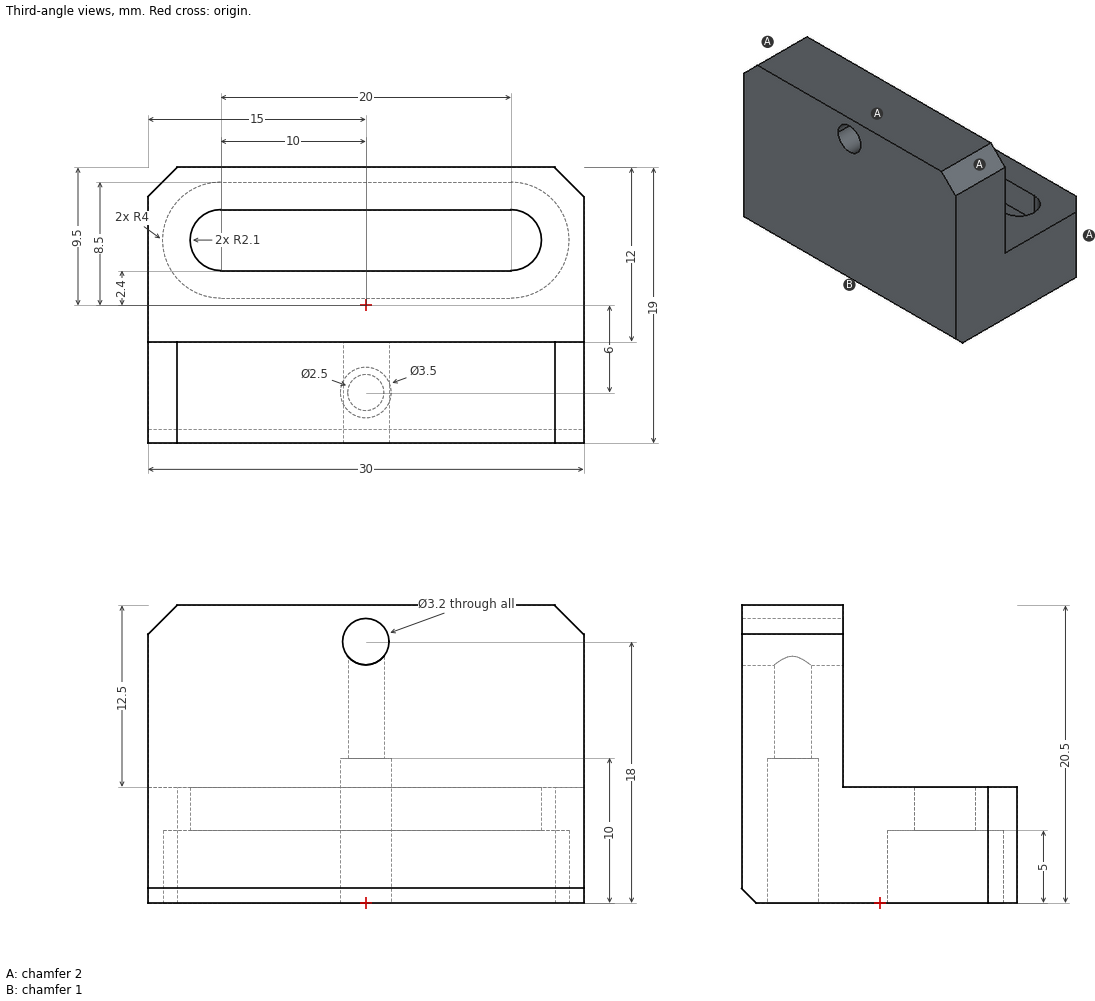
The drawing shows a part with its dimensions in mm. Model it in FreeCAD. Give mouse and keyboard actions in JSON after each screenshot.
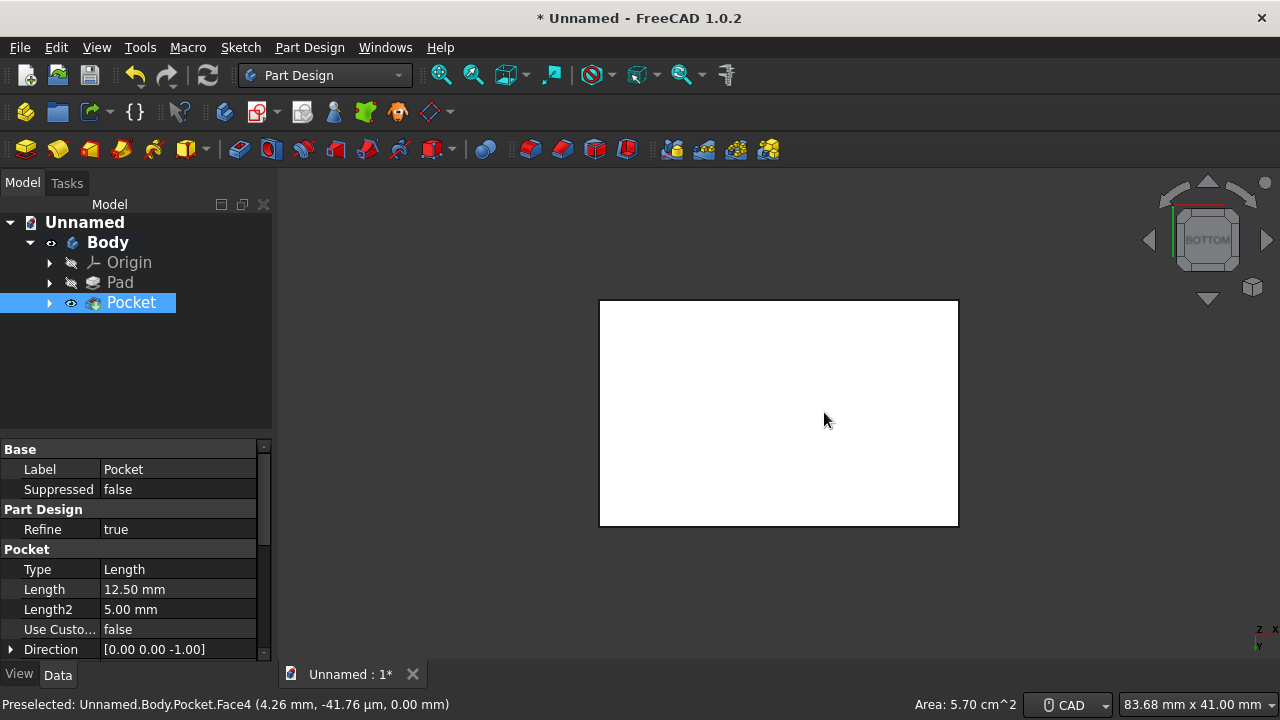
{"action": "left_click", "coordinate": [258, 112]}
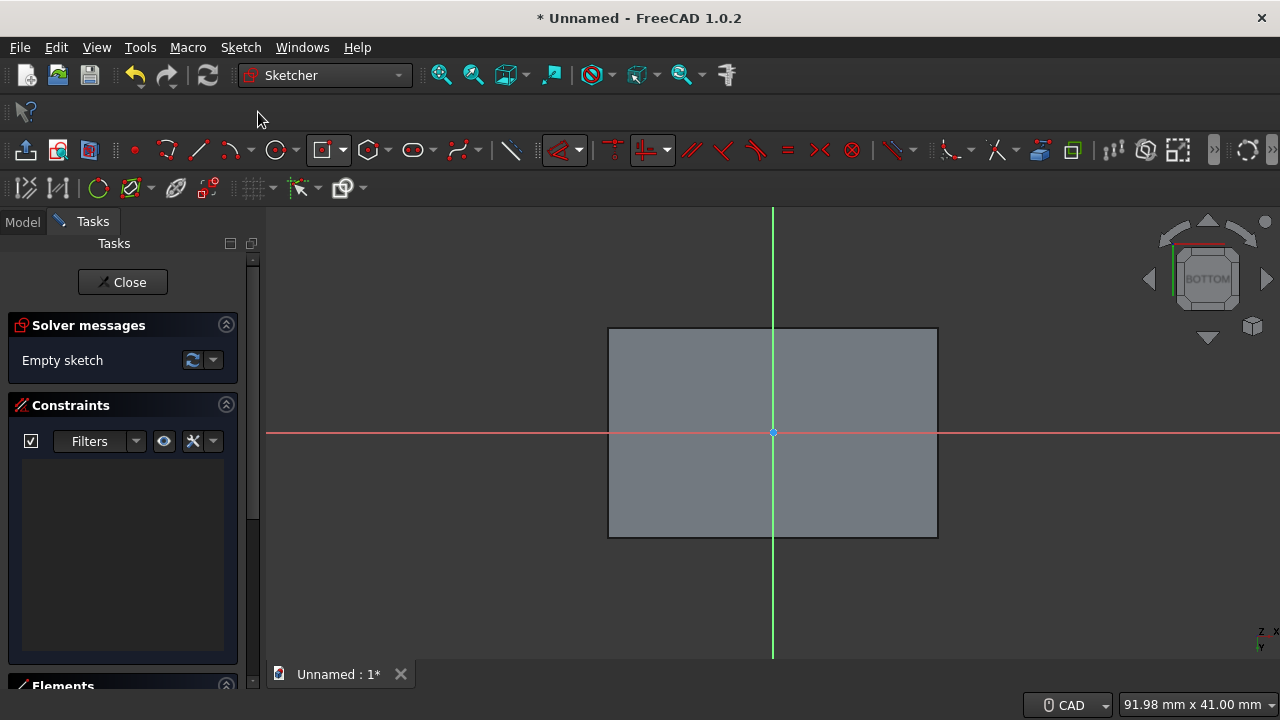
{"action": "scroll", "coordinate": [829, 499], "scroll_direction": "up", "scroll_amount": 4}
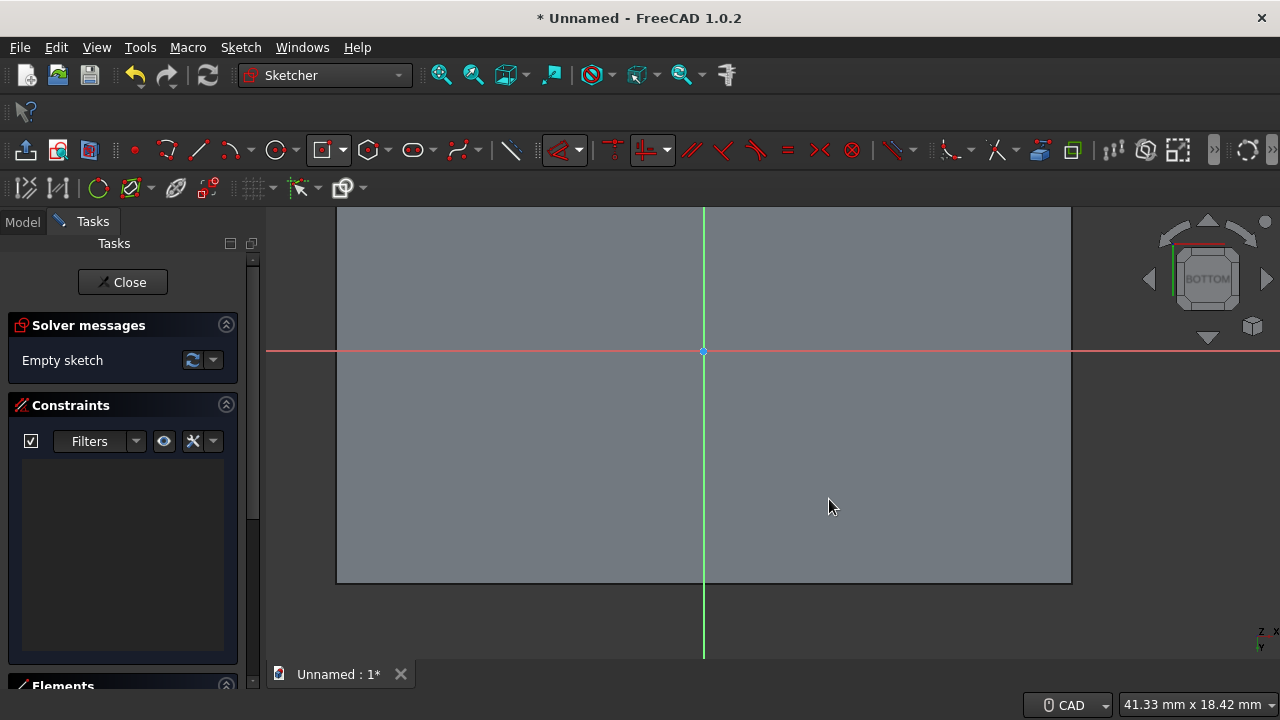
{"action": "left_click", "coordinate": [414, 150]}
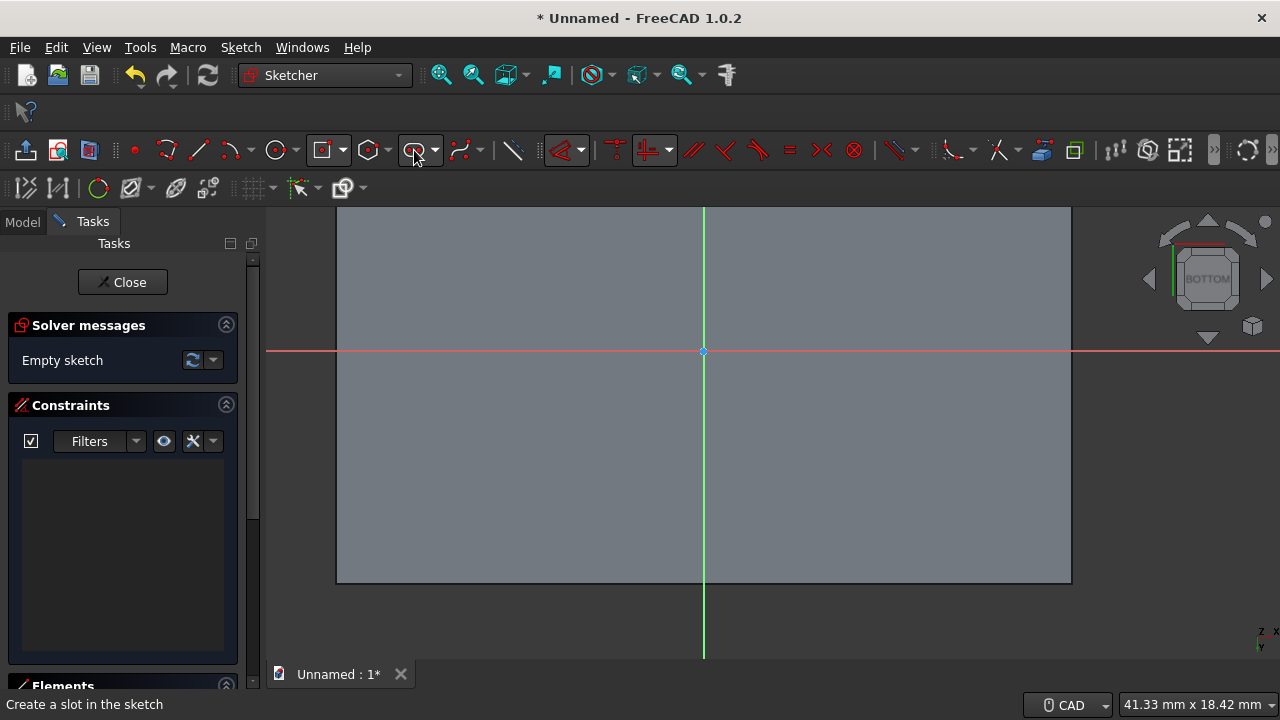
{"action": "left_click", "coordinate": [458, 462]}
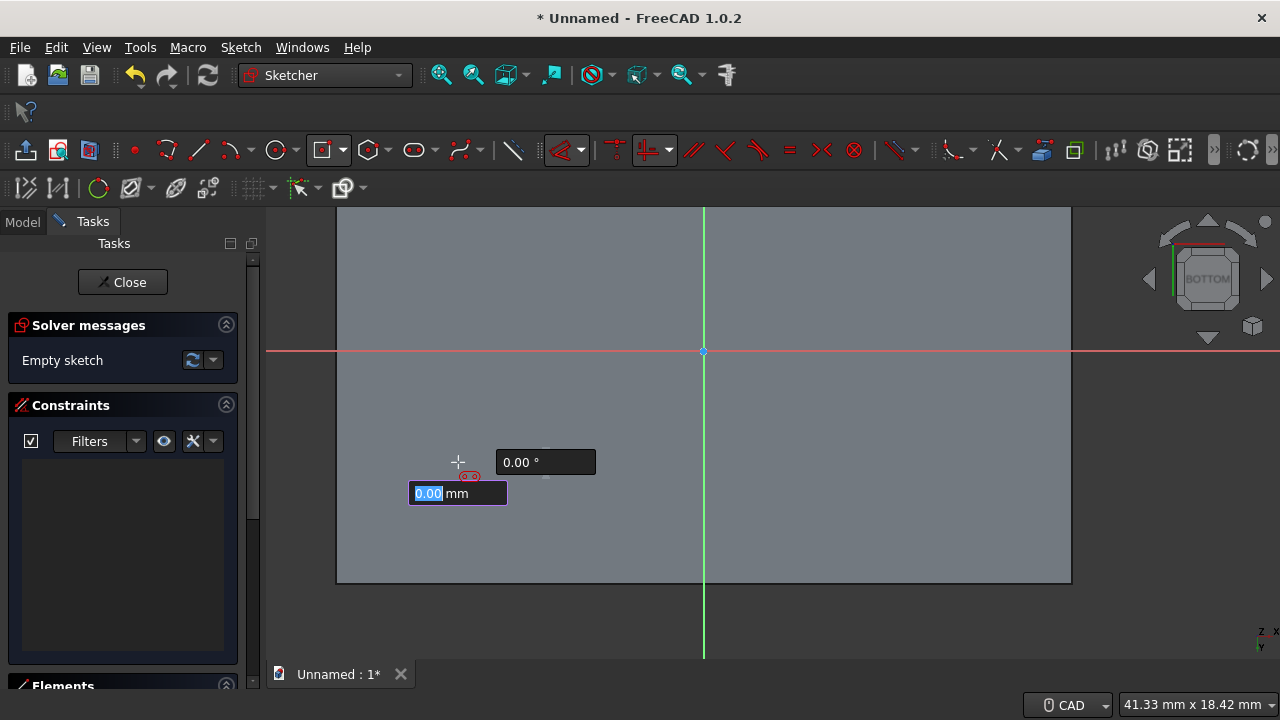
{"action": "left_click", "coordinate": [949, 462]}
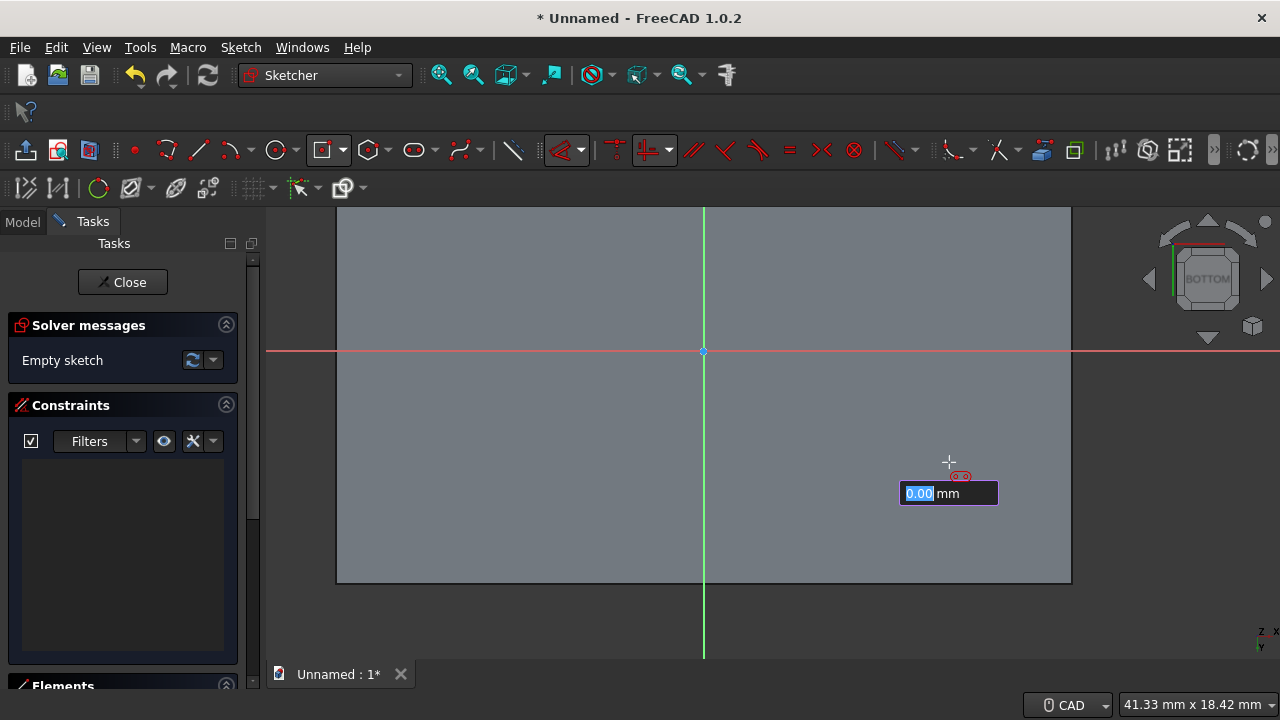
{"action": "left_click", "coordinate": [777, 410]}
{"action": "key", "text": "Escape"}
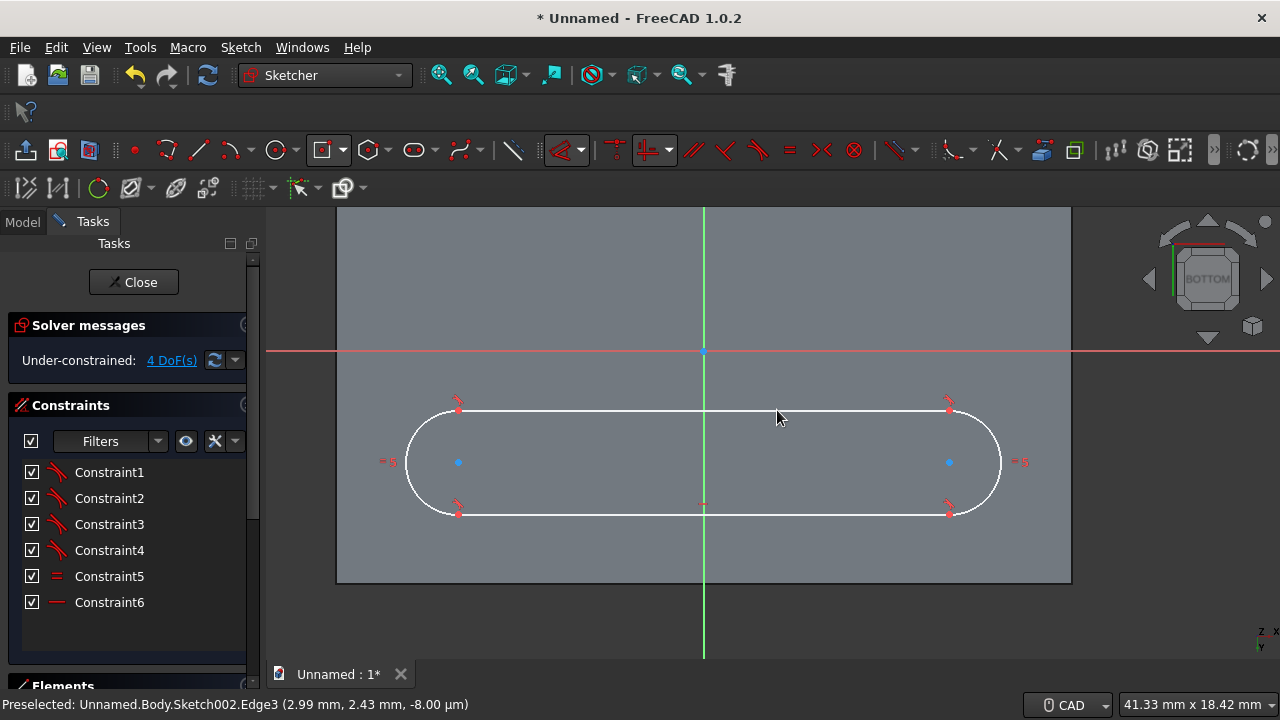
{"action": "left_click", "coordinate": [416, 432]}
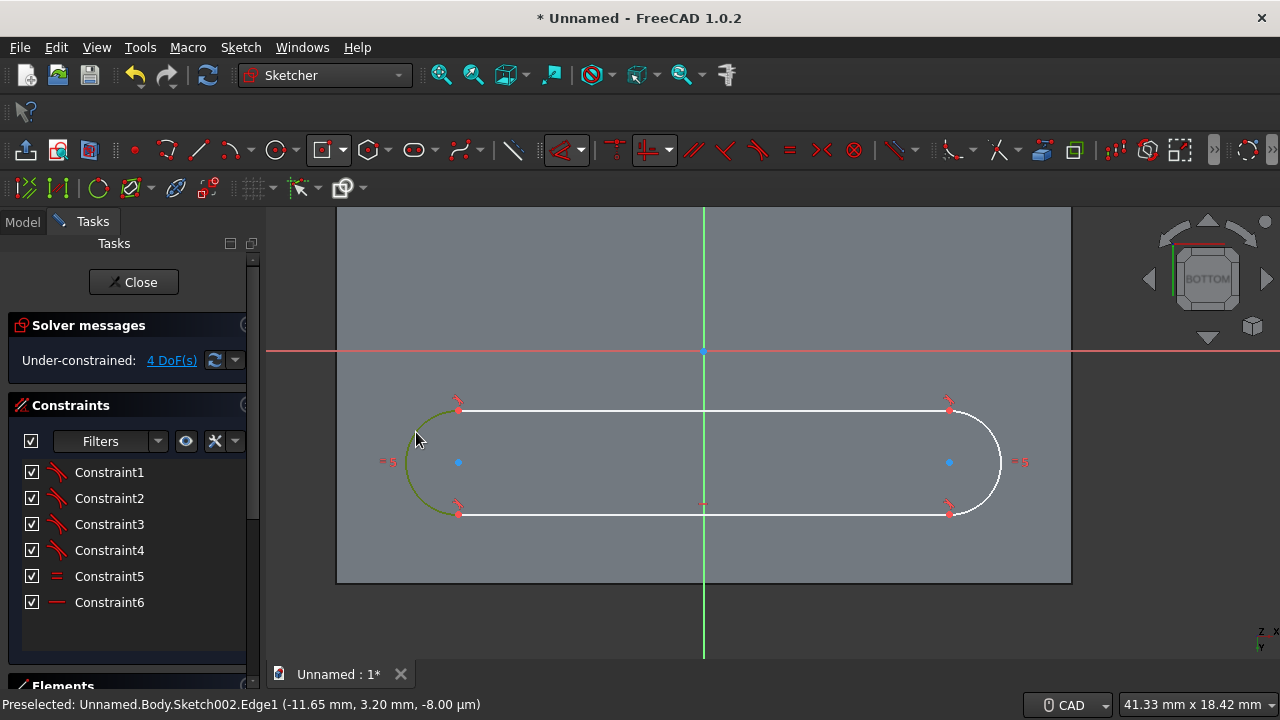
{"action": "key", "text": "k r"}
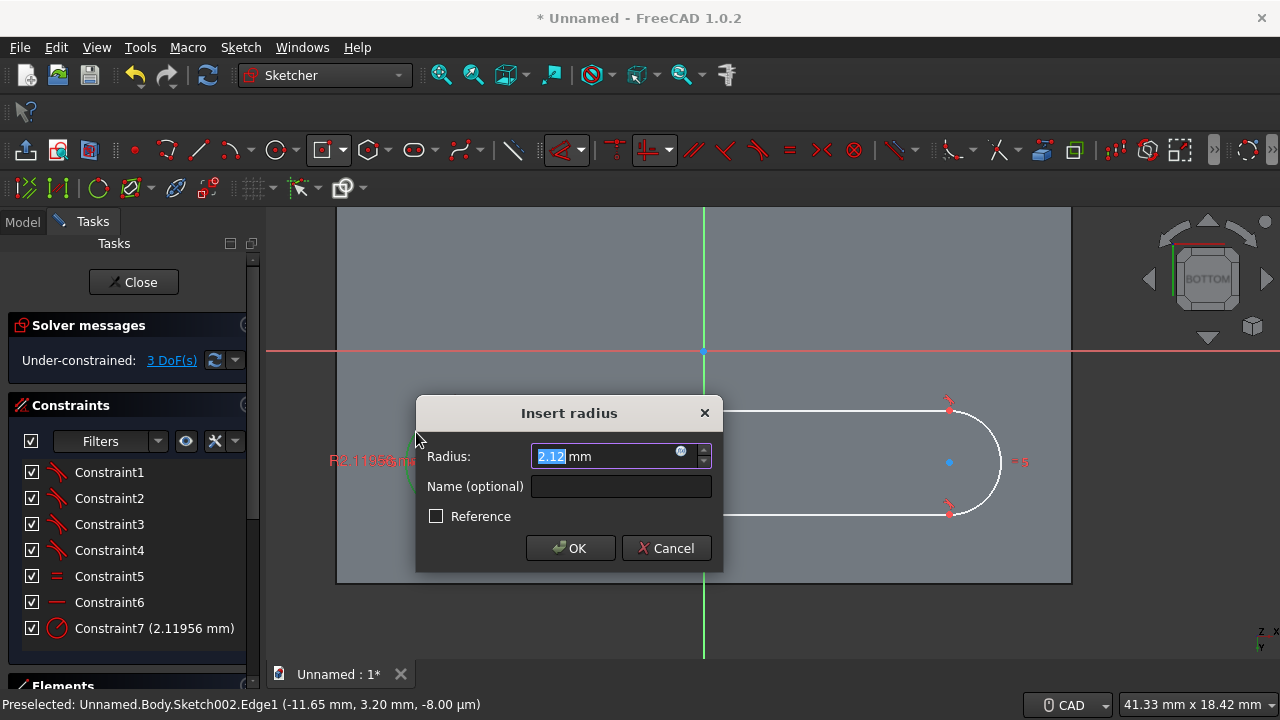
{"action": "type", "text": "2.1"}
{"action": "key", "text": "Return"}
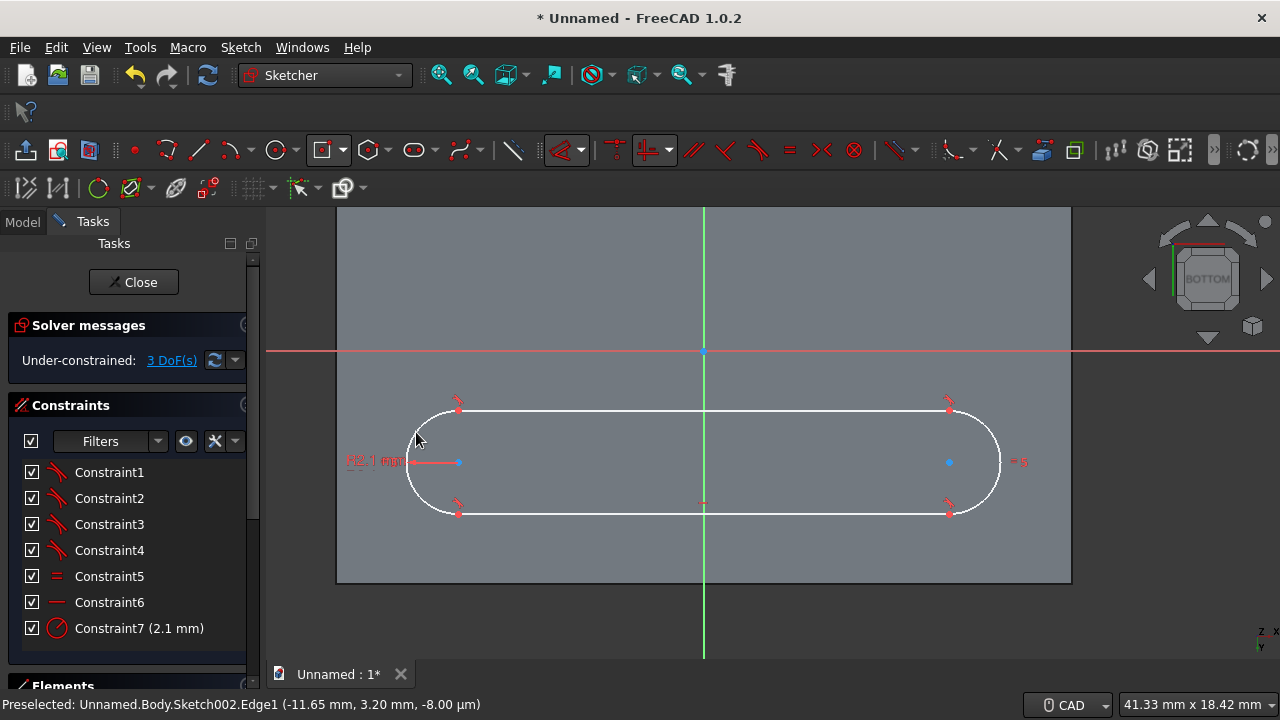
{"action": "left_click", "coordinate": [605, 411]}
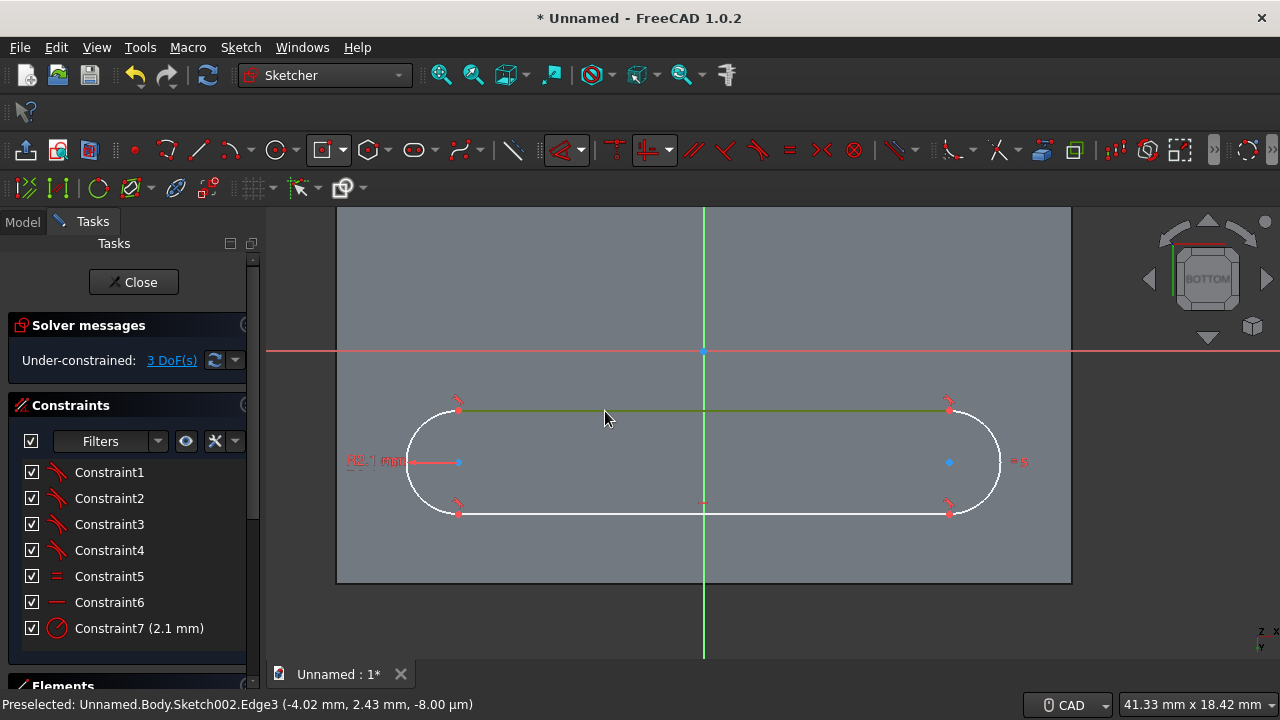
{"action": "left_click", "coordinate": [584, 150]}